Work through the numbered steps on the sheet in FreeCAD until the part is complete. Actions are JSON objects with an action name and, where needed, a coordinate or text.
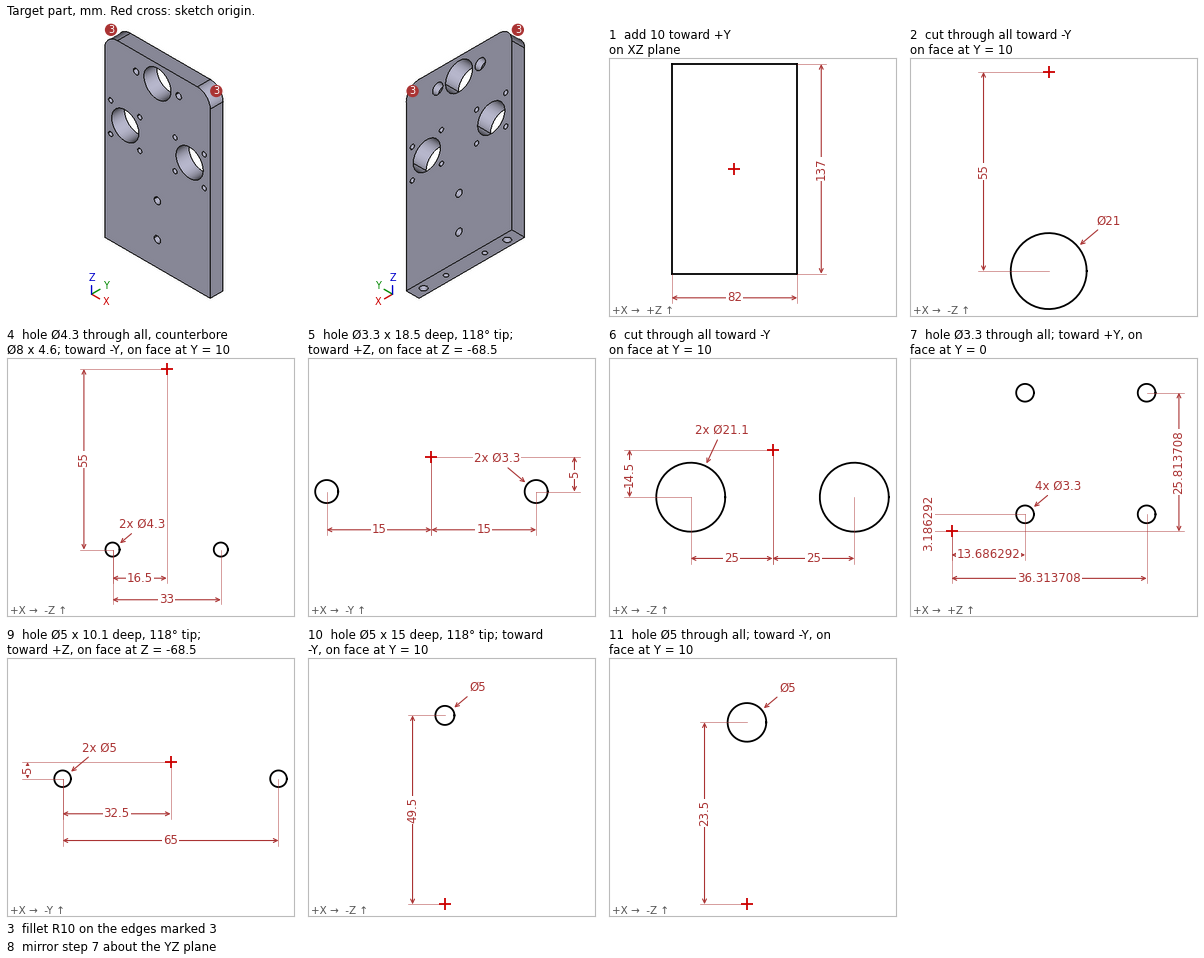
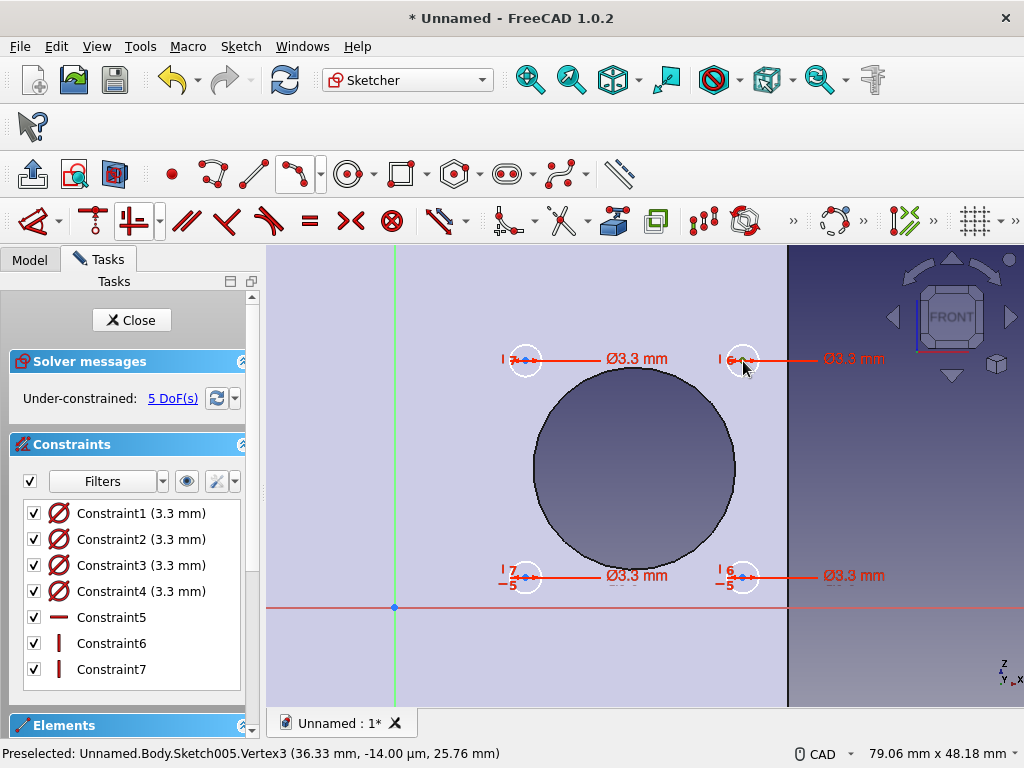
{"action": "left_click", "coordinate": [526, 361]}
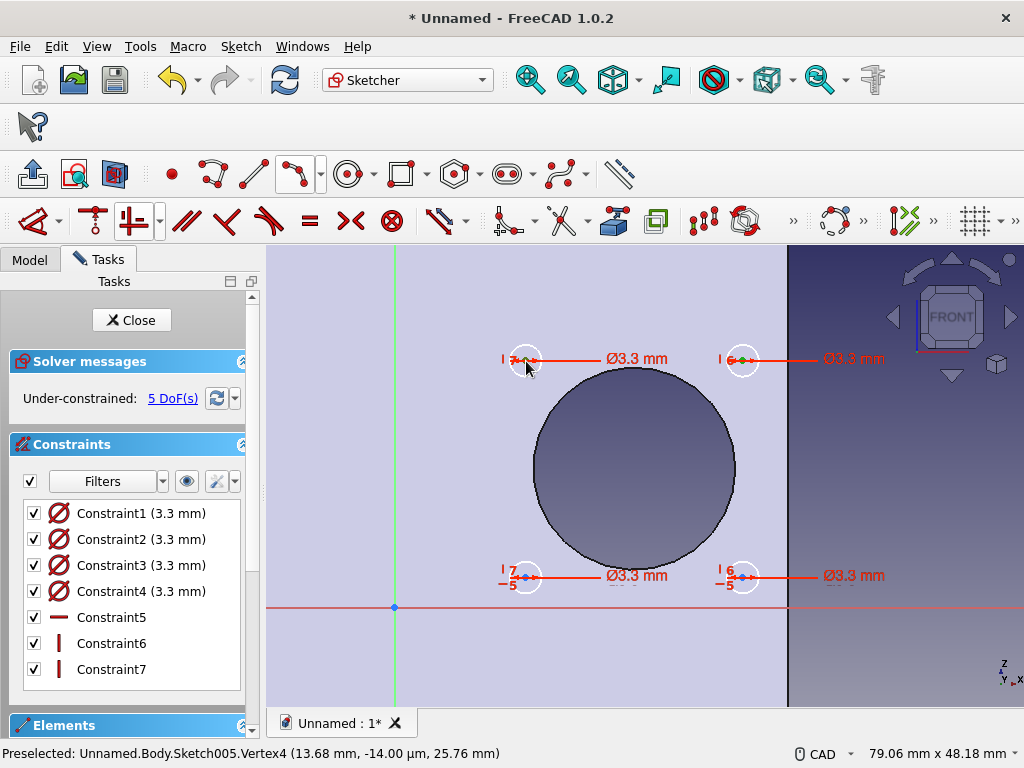
{"action": "left_click", "coordinate": [160, 222]}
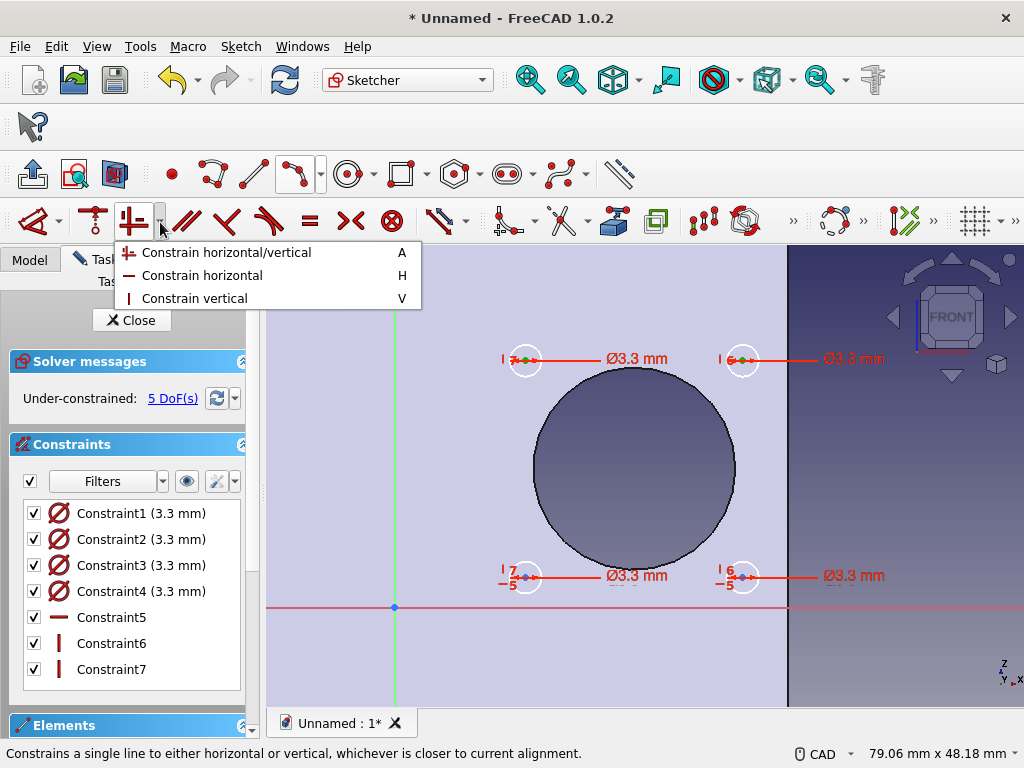
{"action": "left_click", "coordinate": [268, 276]}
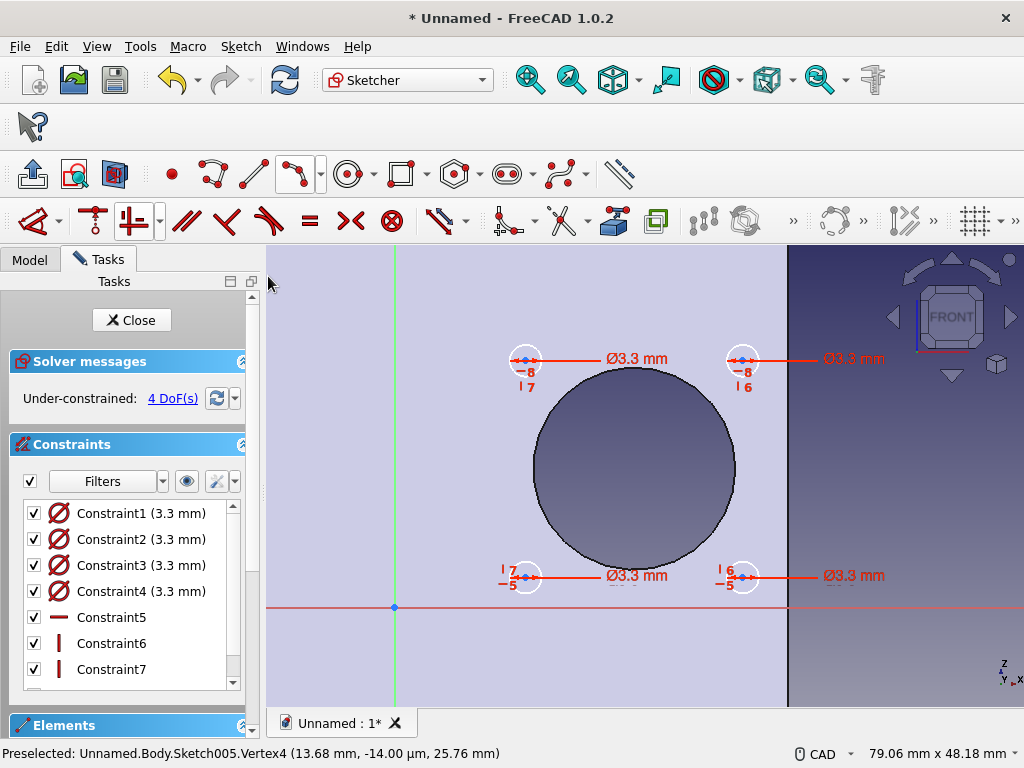
{"action": "key", "text": "d"}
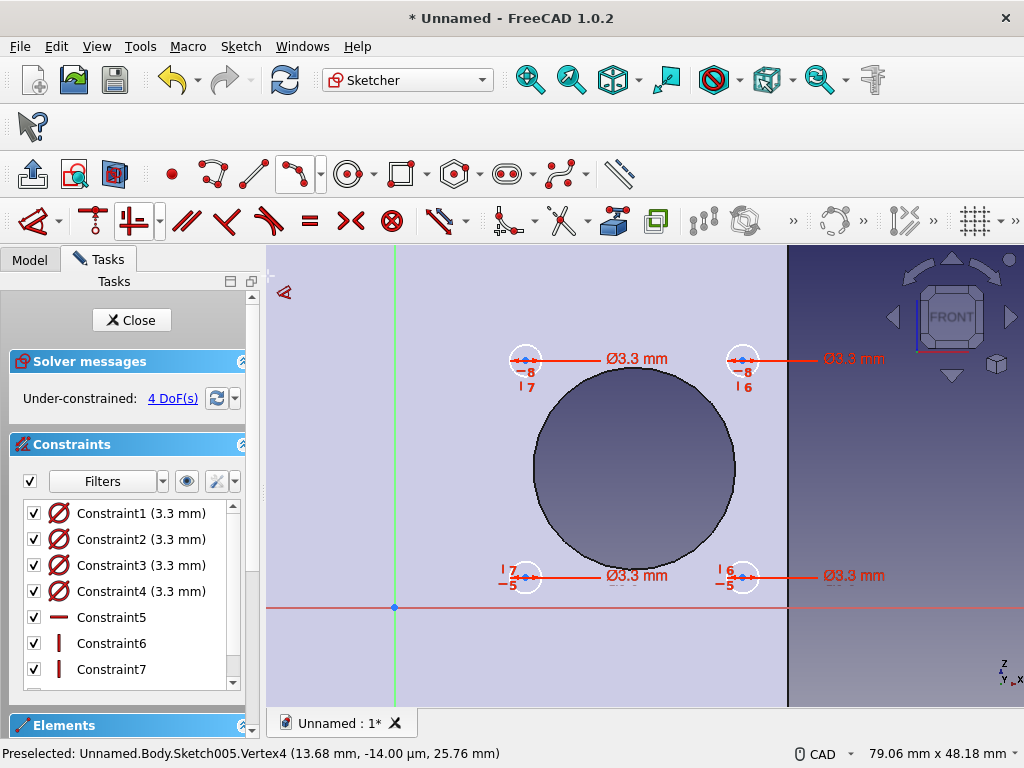
{"action": "scroll", "coordinate": [526, 578], "scroll_direction": "up", "scroll_amount": 2}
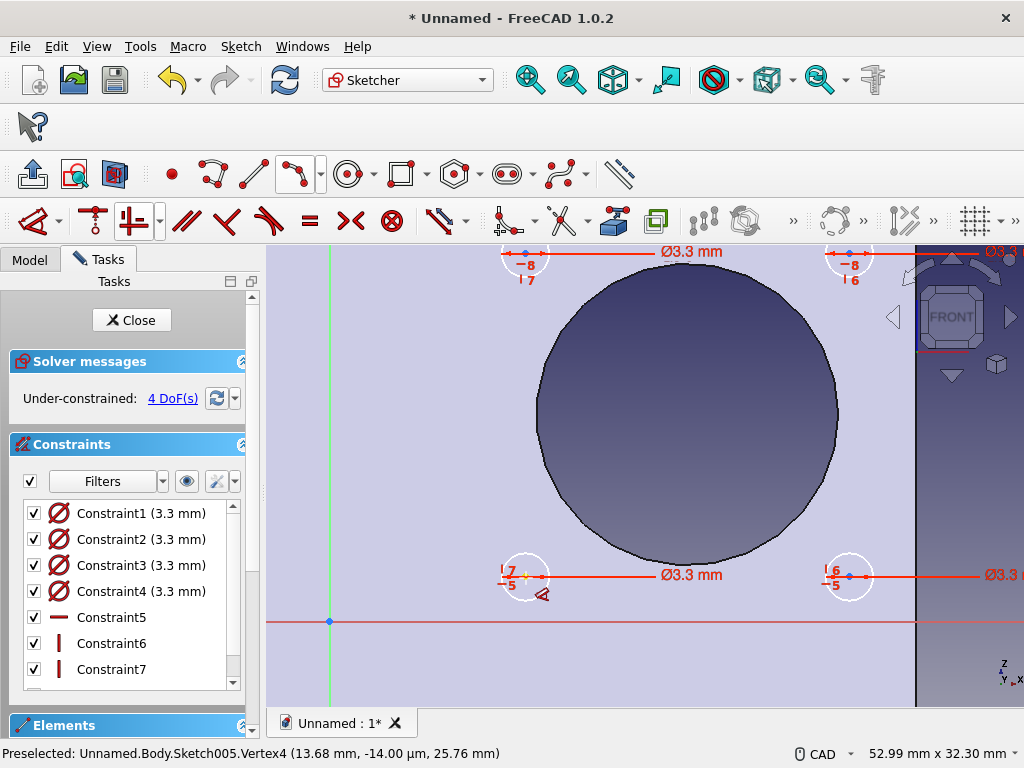
{"action": "left_click", "coordinate": [525, 577]}
{"action": "left_click", "coordinate": [296, 599]}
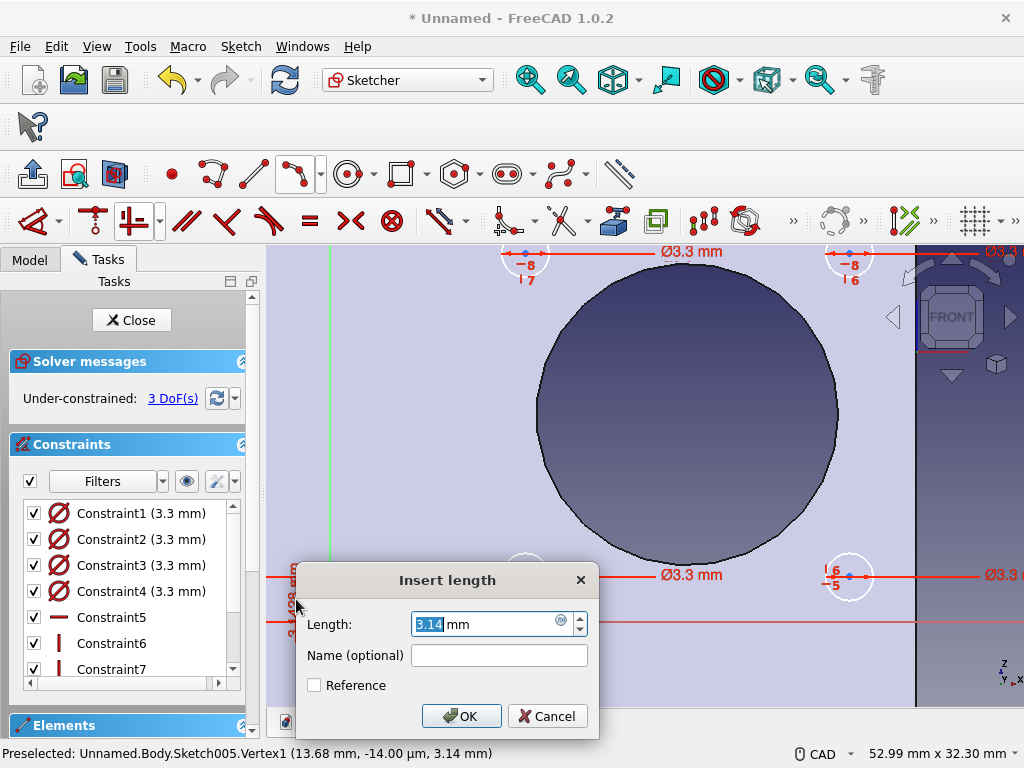
{"action": "type", "text": "3.186292"}
{"action": "key", "text": "Return"}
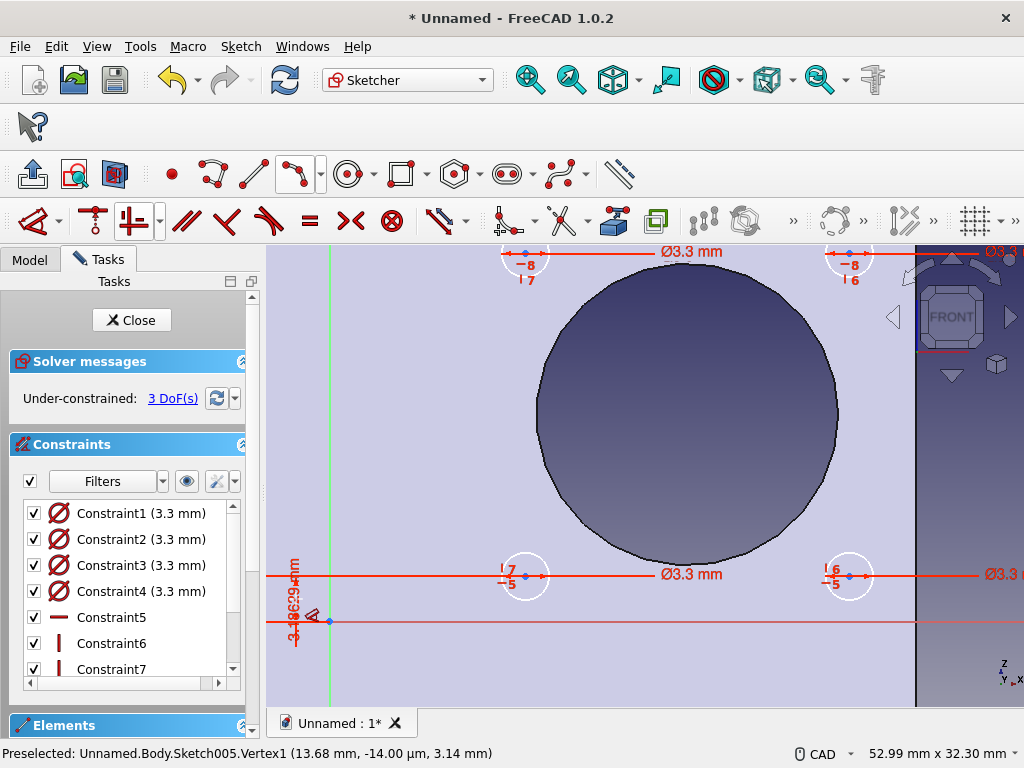
{"action": "left_click", "coordinate": [525, 576]}
{"action": "left_click", "coordinate": [428, 656]}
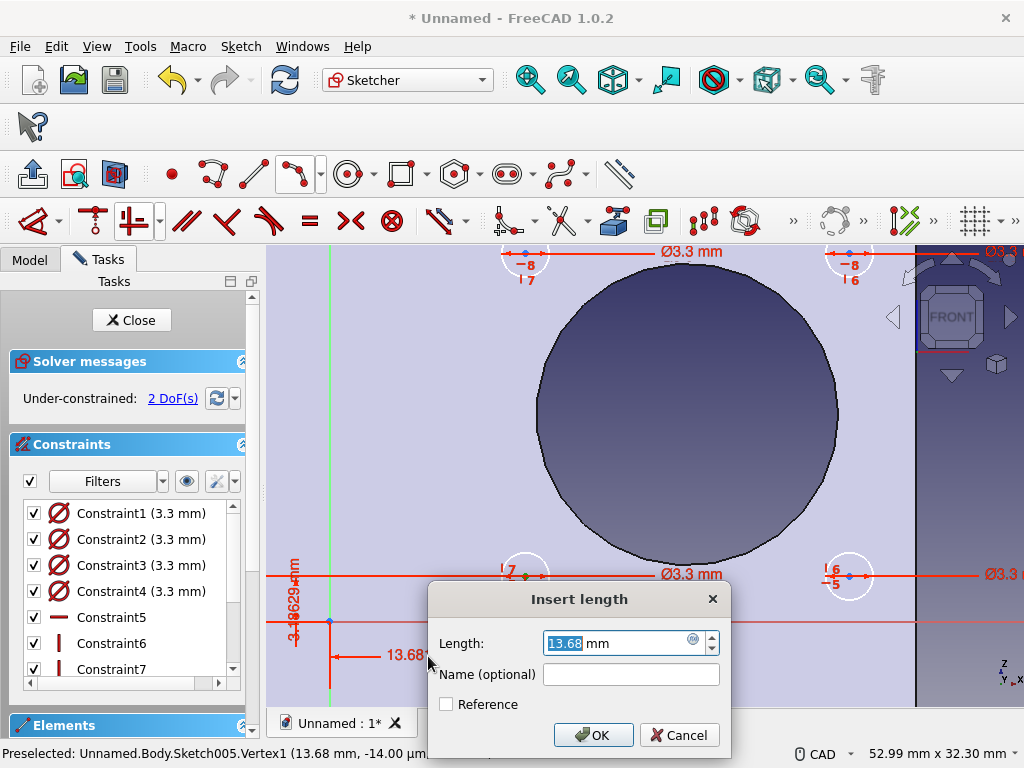
{"action": "type", "text": "13.686292"}
{"action": "key", "text": "Return"}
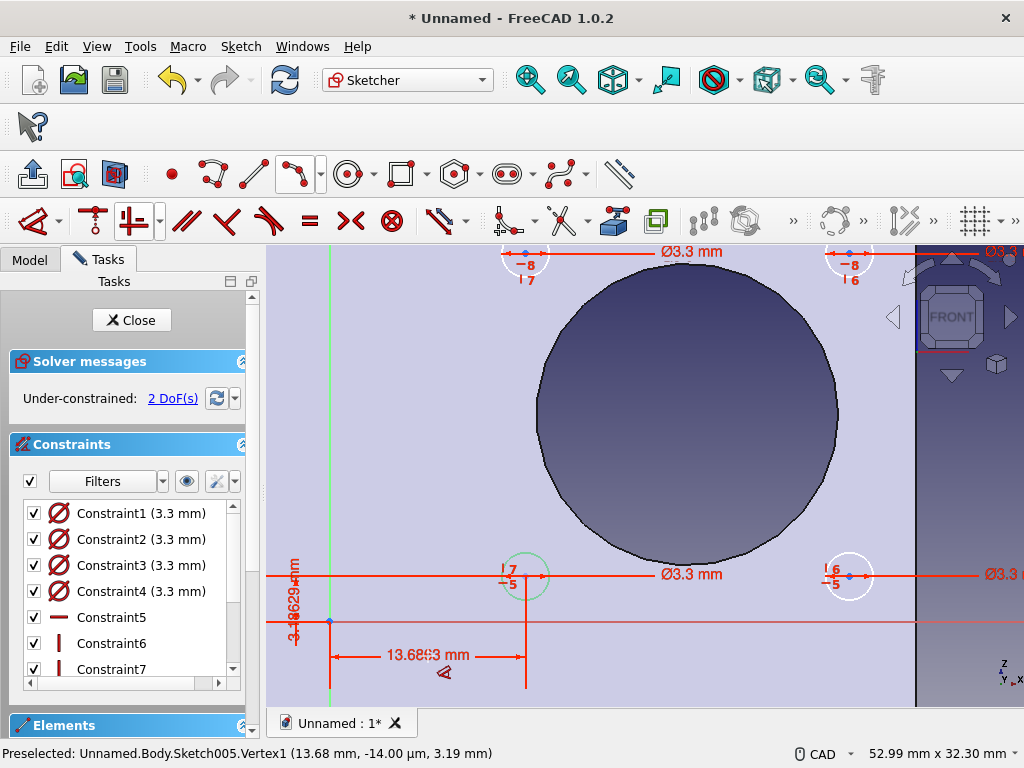
{"action": "left_click", "coordinate": [849, 576]}
{"action": "left_click", "coordinate": [590, 656]}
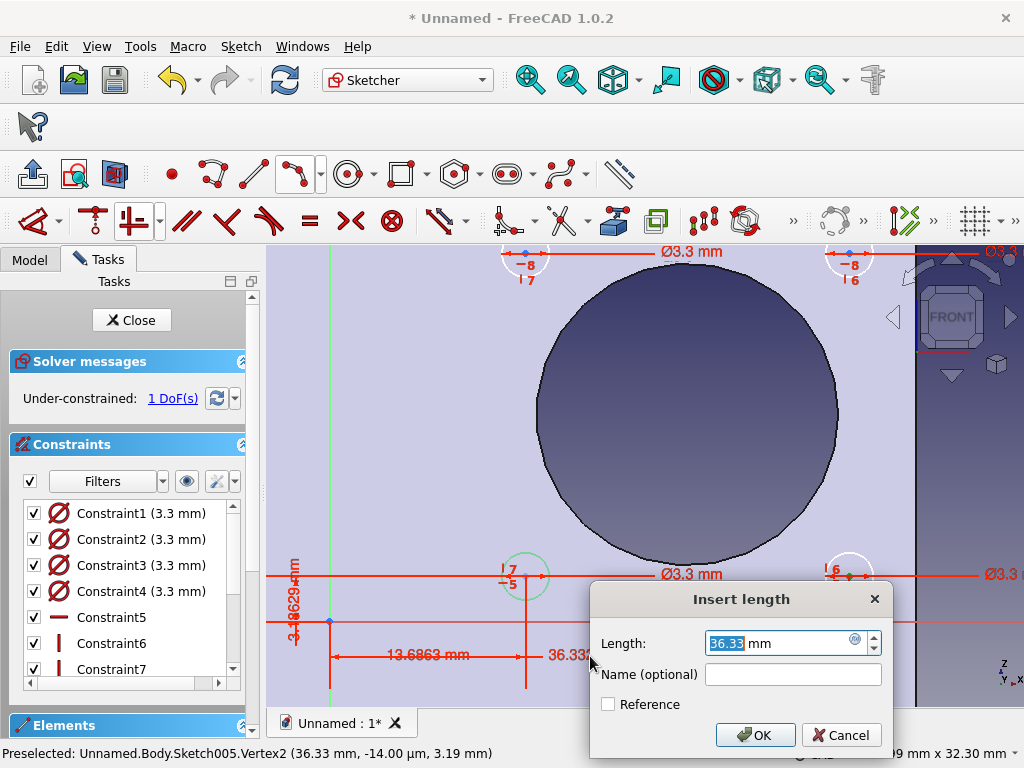
{"action": "type", "text": "36.313708"}
{"action": "key", "text": "Return"}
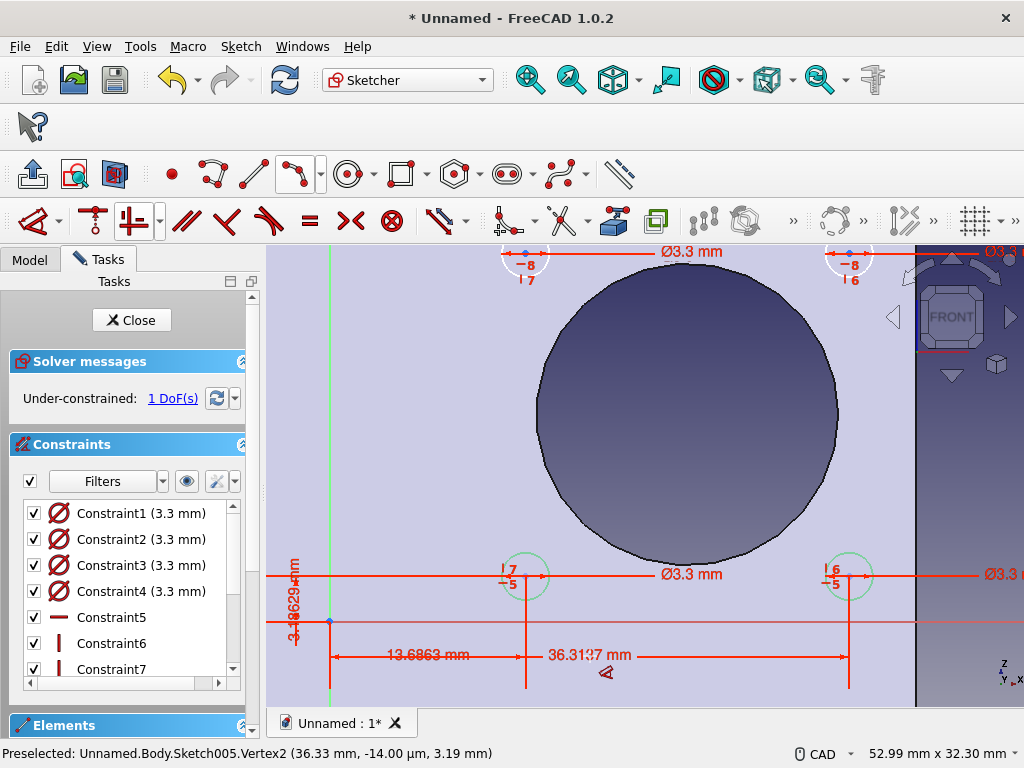
{"action": "scroll", "coordinate": [526, 579], "scroll_direction": "down", "scroll_amount": 2}